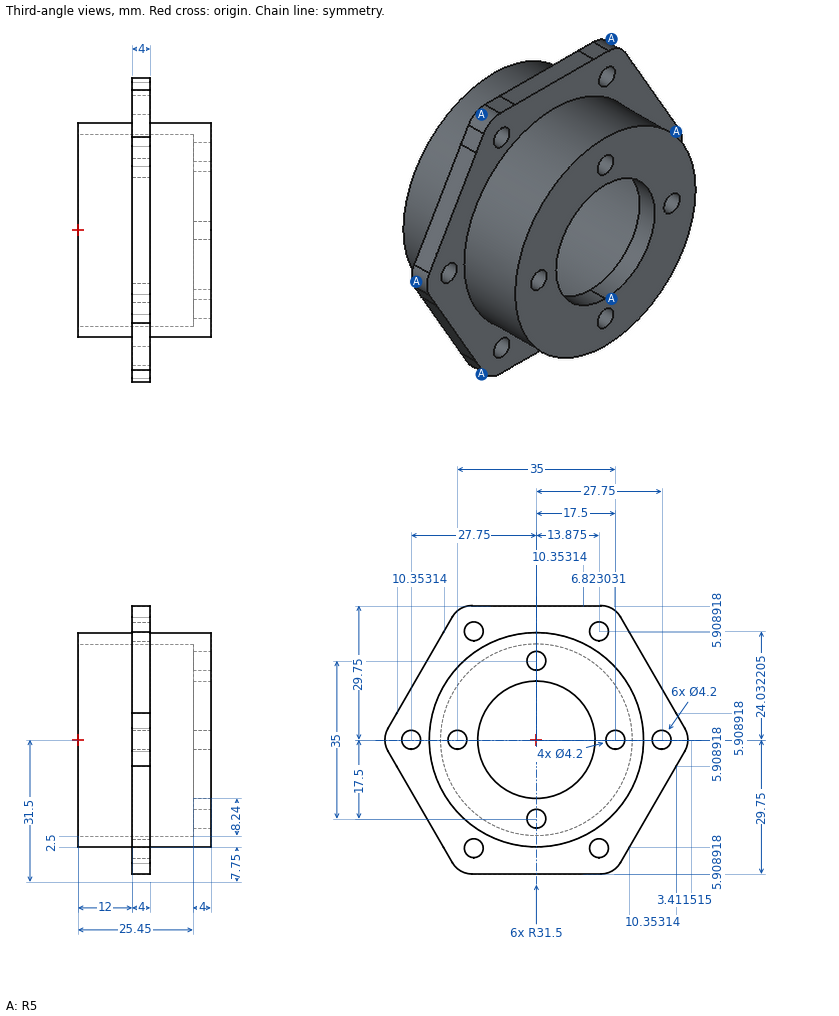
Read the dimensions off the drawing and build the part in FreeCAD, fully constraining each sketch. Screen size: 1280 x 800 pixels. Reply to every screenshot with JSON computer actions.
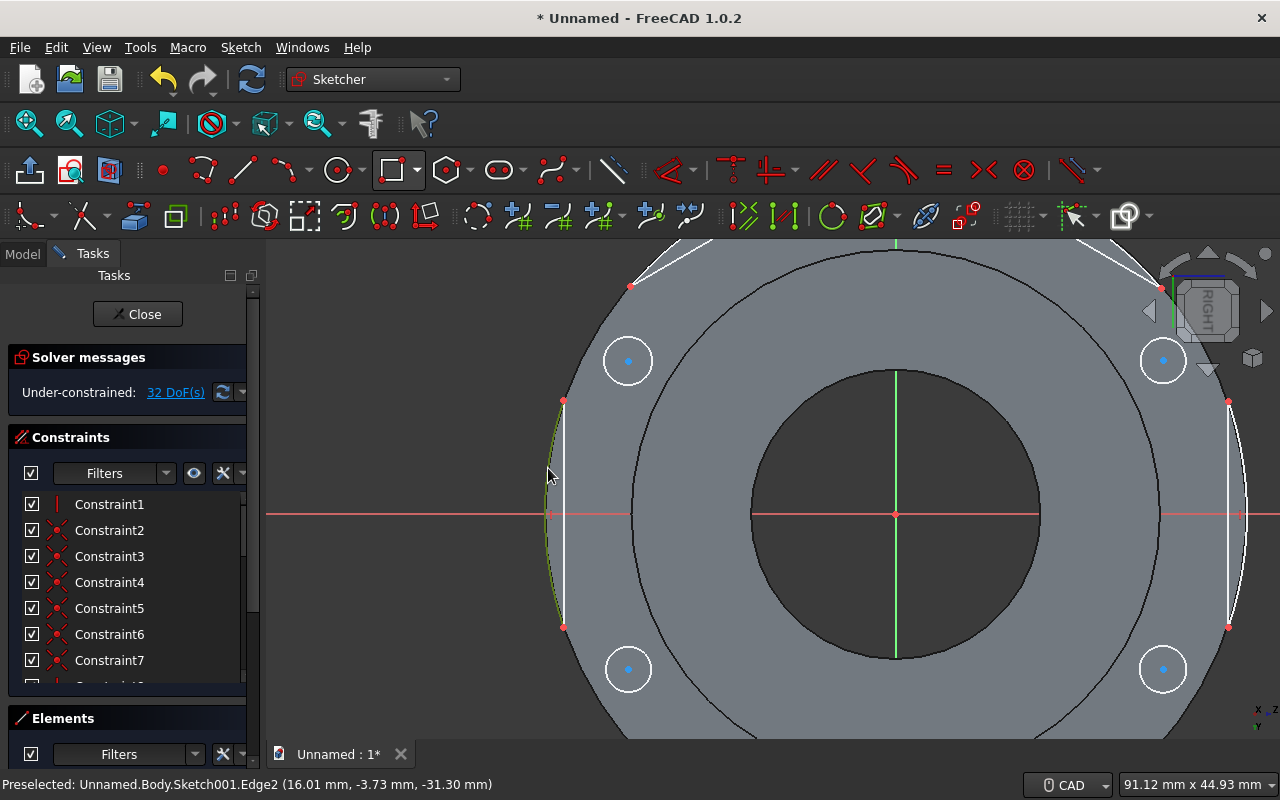
{"action": "scroll", "coordinate": [548, 468], "scroll_direction": "down", "scroll_amount": 4}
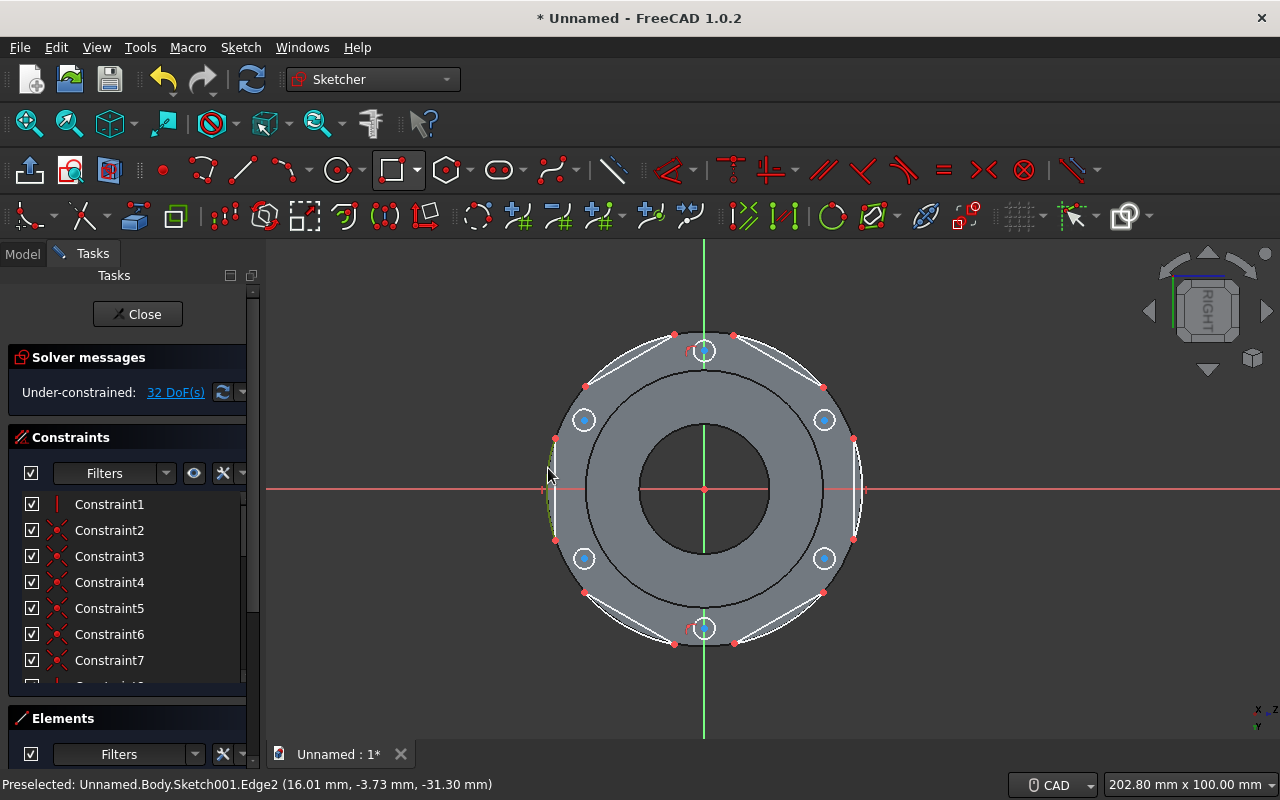
{"action": "scroll", "coordinate": [608, 614], "scroll_direction": "up", "scroll_amount": 4}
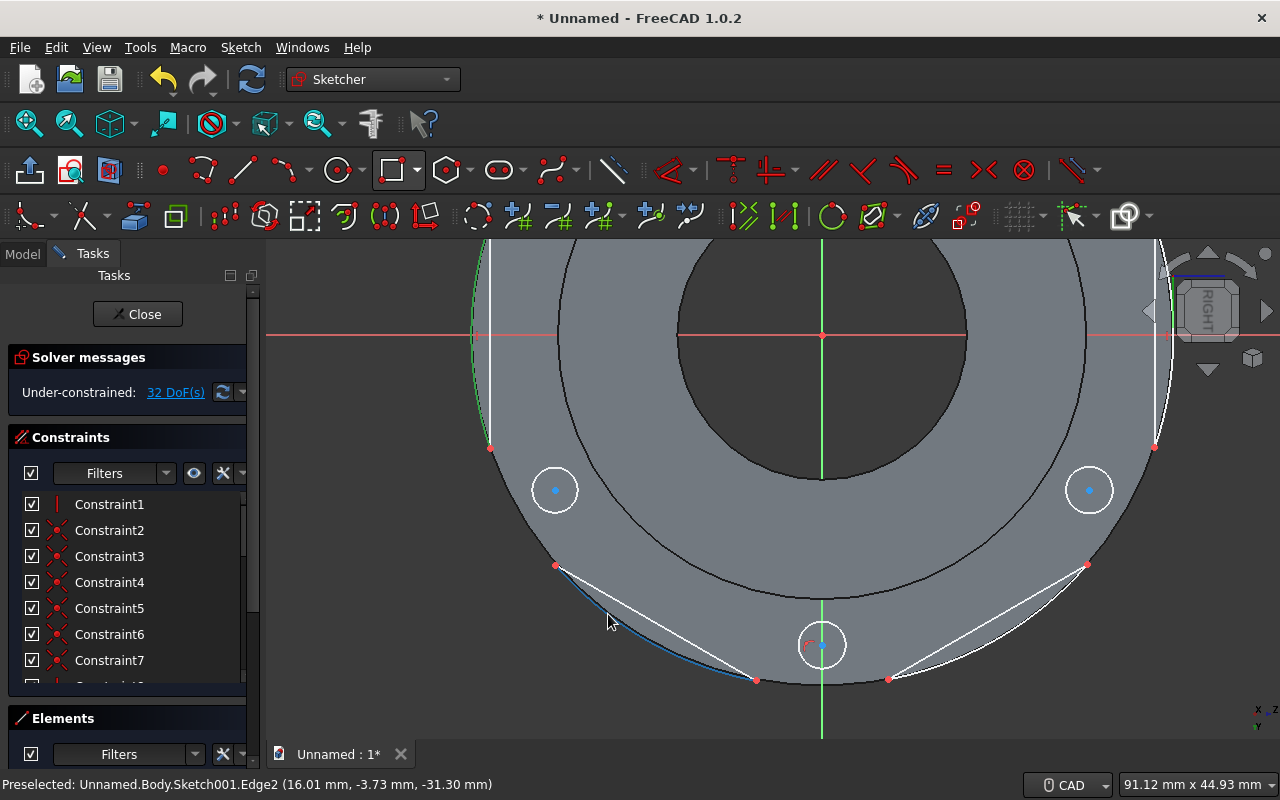
{"action": "left_click", "coordinate": [607, 614]}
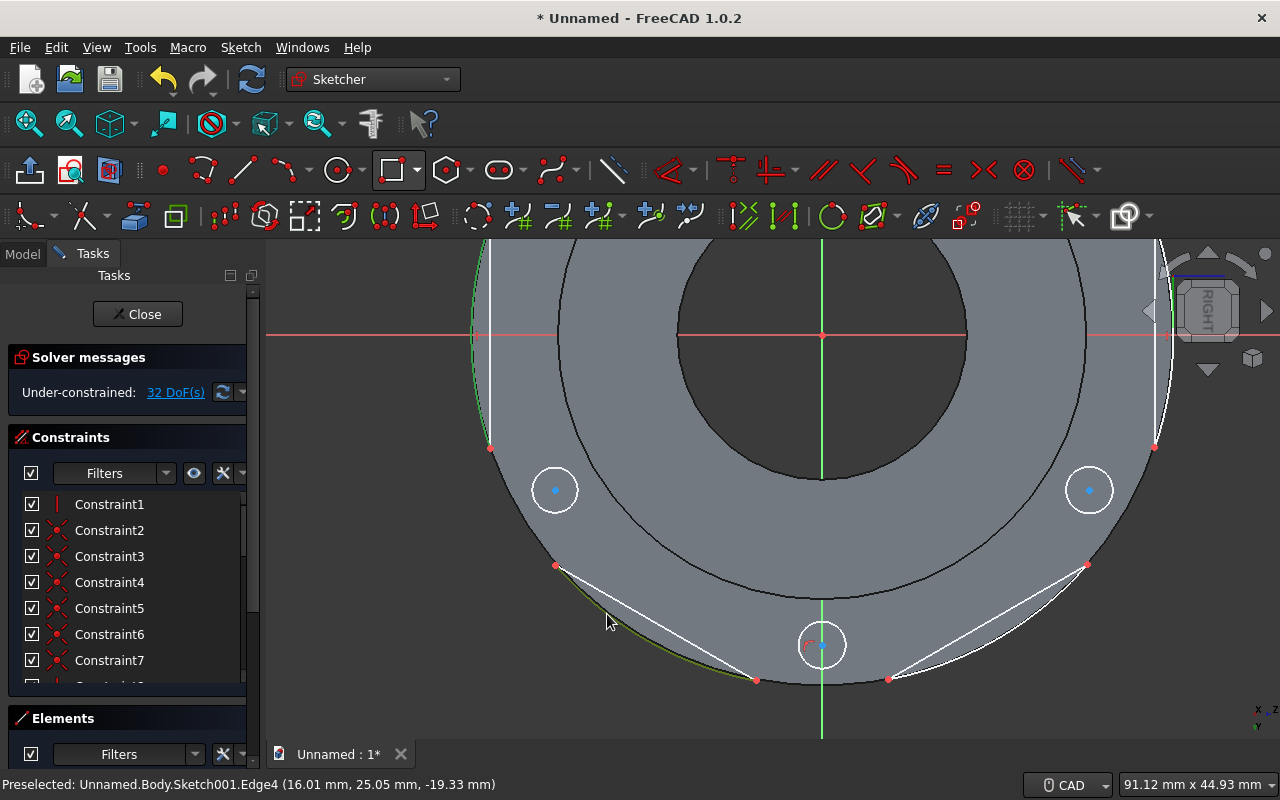
{"action": "left_click", "coordinate": [955, 660]}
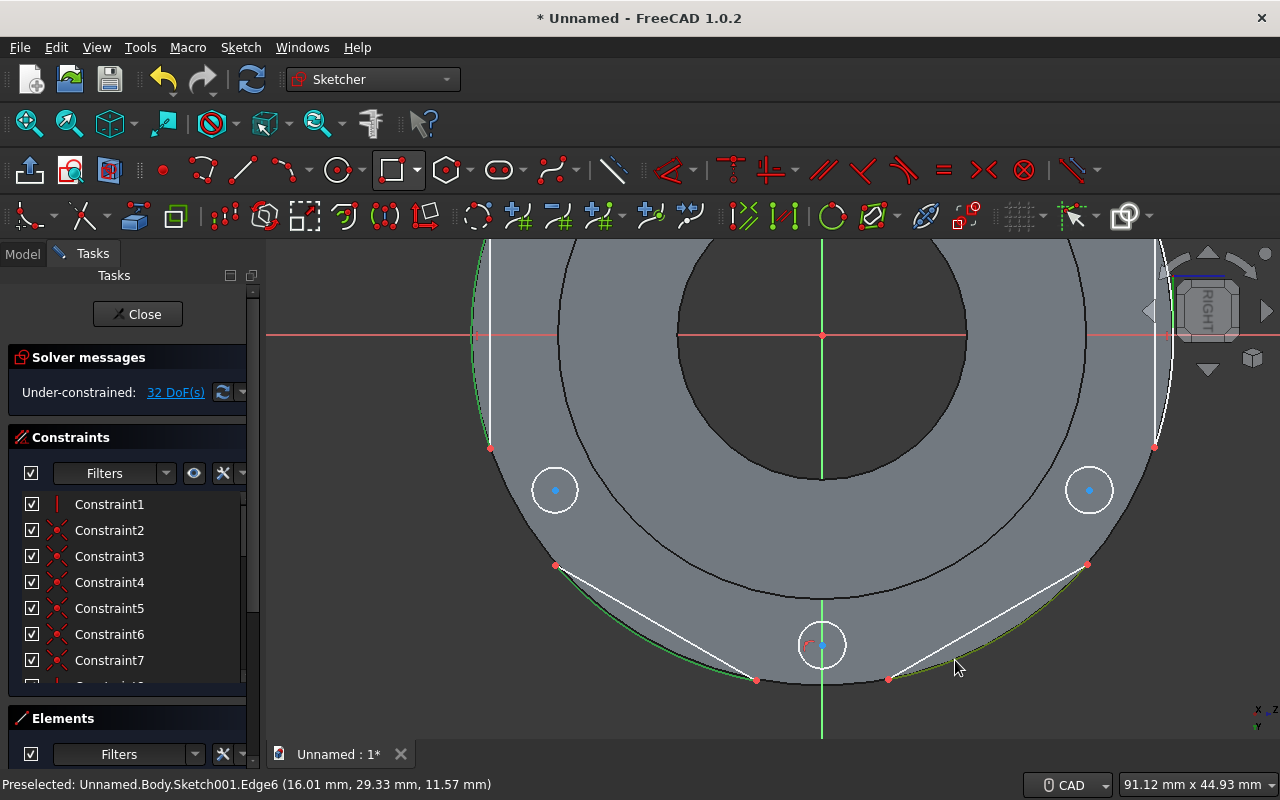
{"action": "scroll", "coordinate": [609, 615], "scroll_direction": "down", "scroll_amount": 4}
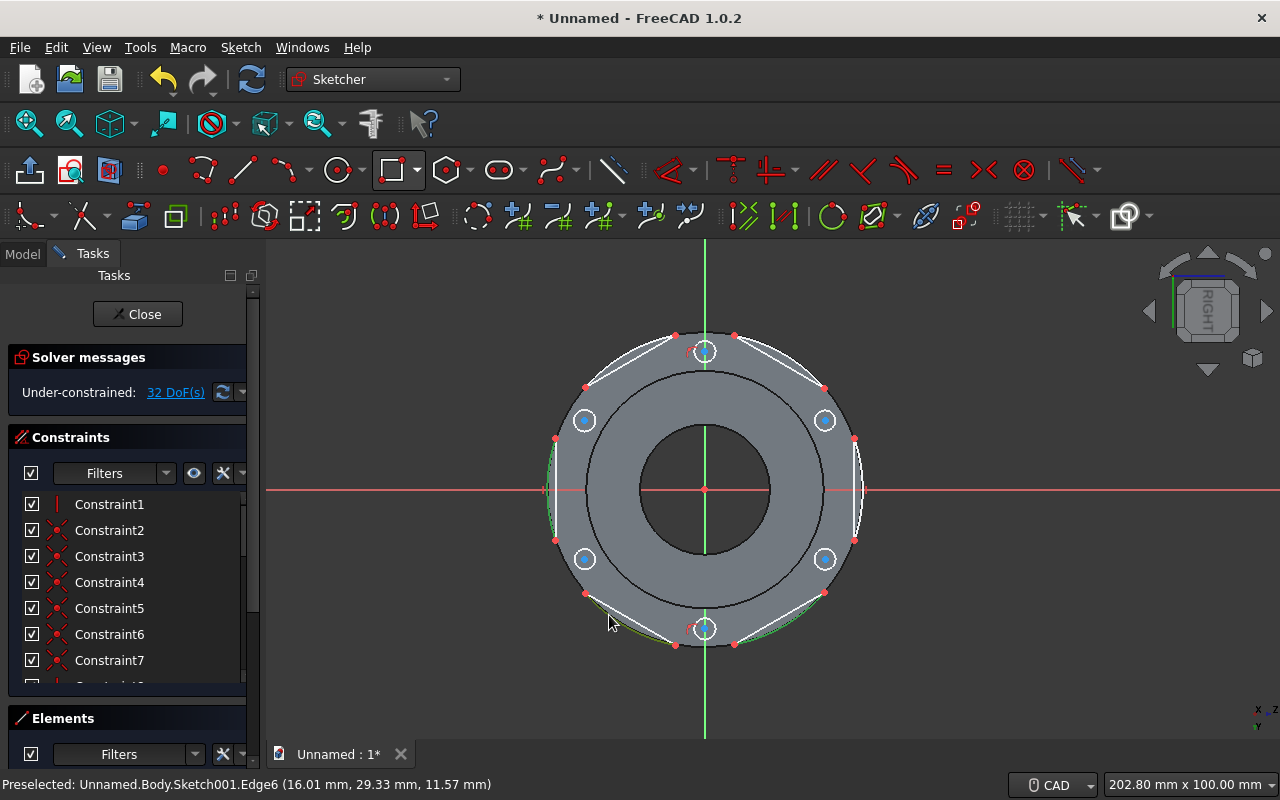
{"action": "scroll", "coordinate": [861, 510], "scroll_direction": "up", "scroll_amount": 4}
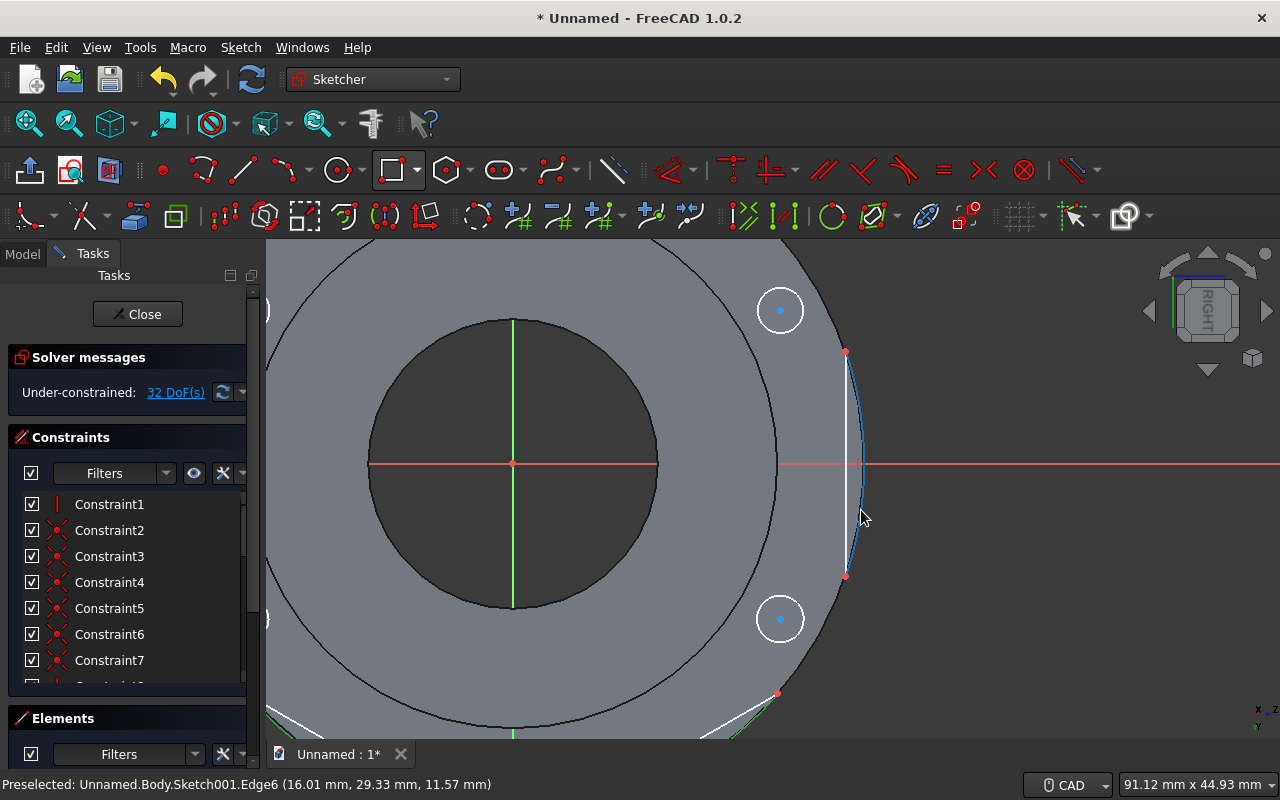
{"action": "left_click", "coordinate": [861, 510]}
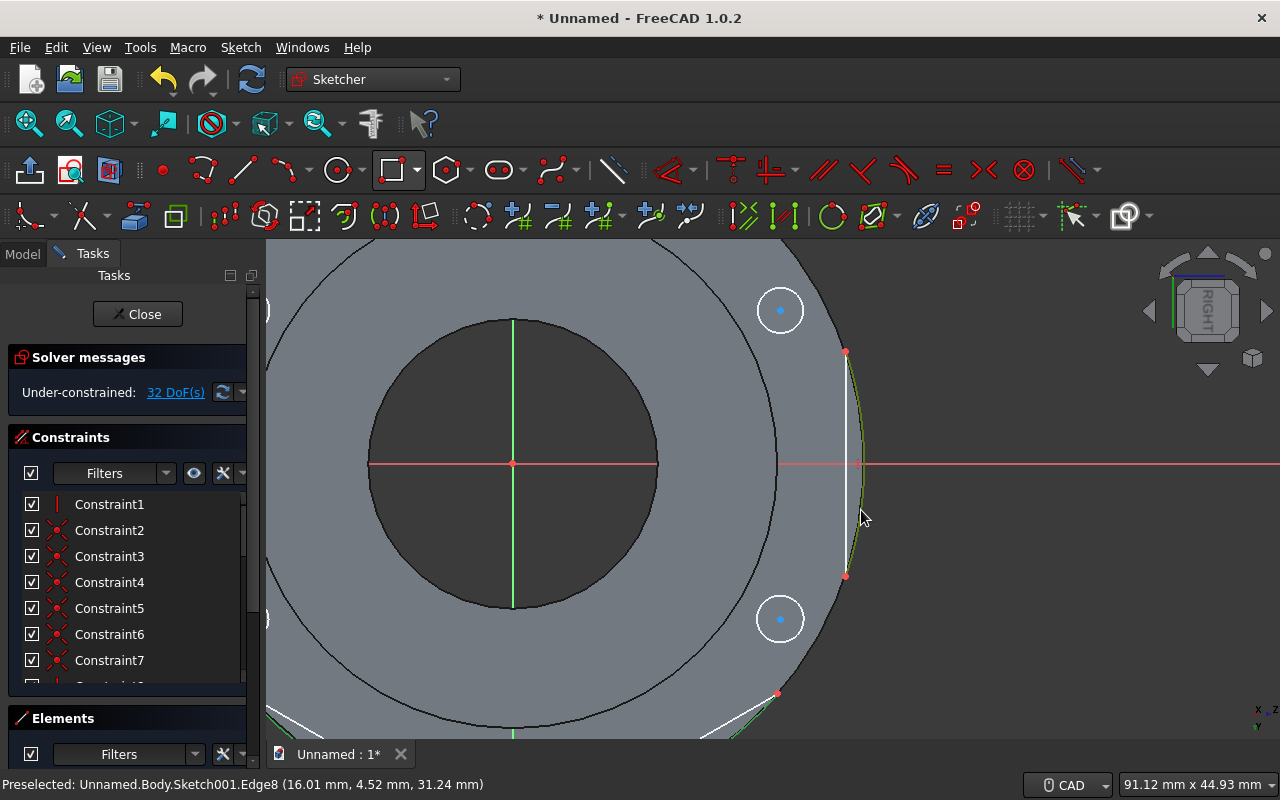
{"action": "scroll", "coordinate": [861, 509], "scroll_direction": "down", "scroll_amount": 4}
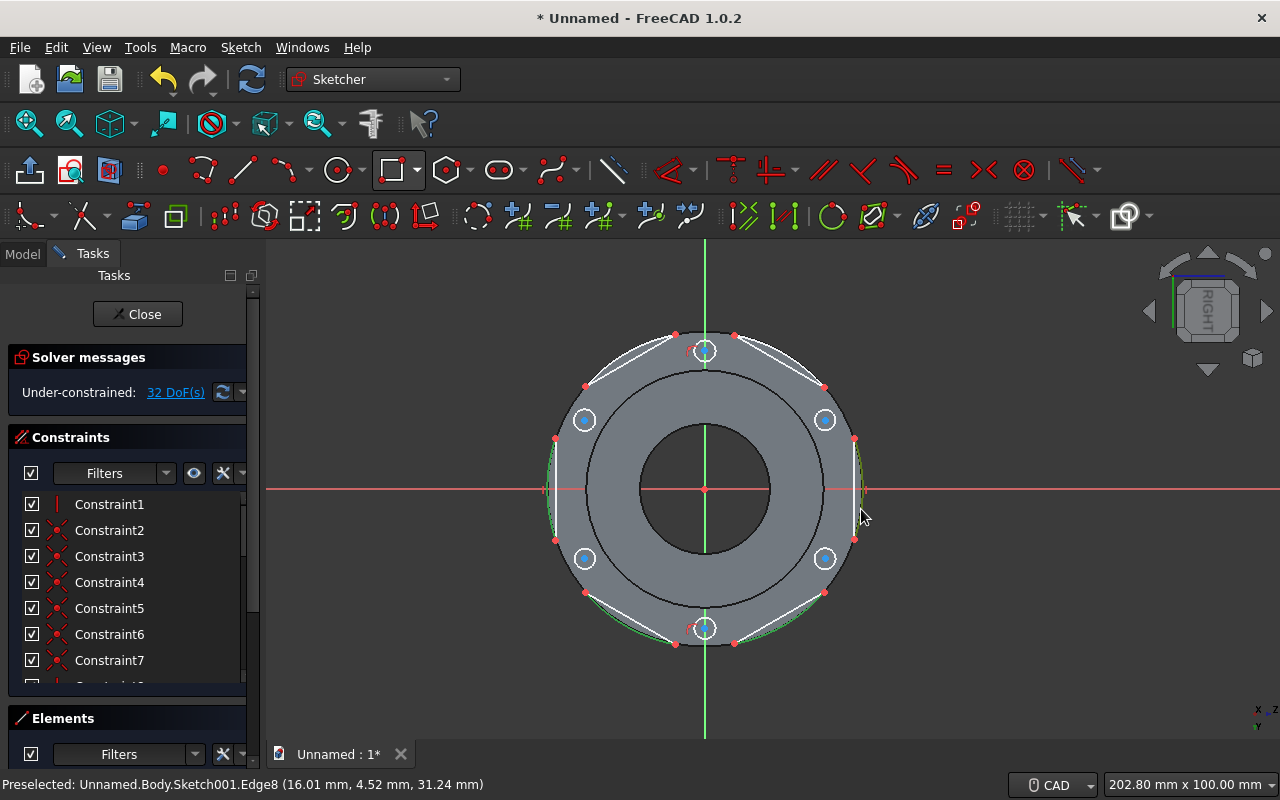
{"action": "scroll", "coordinate": [801, 366], "scroll_direction": "up", "scroll_amount": 4}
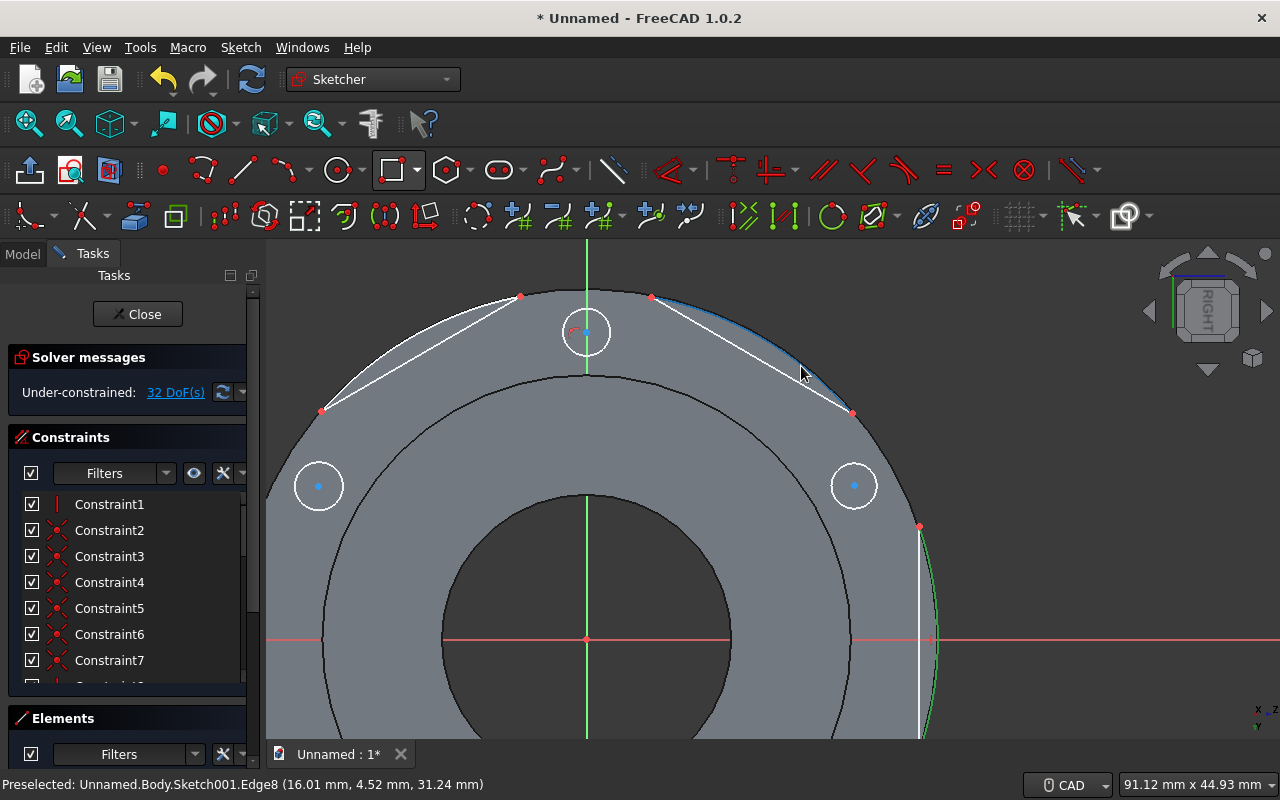
{"action": "left_click", "coordinate": [801, 365]}